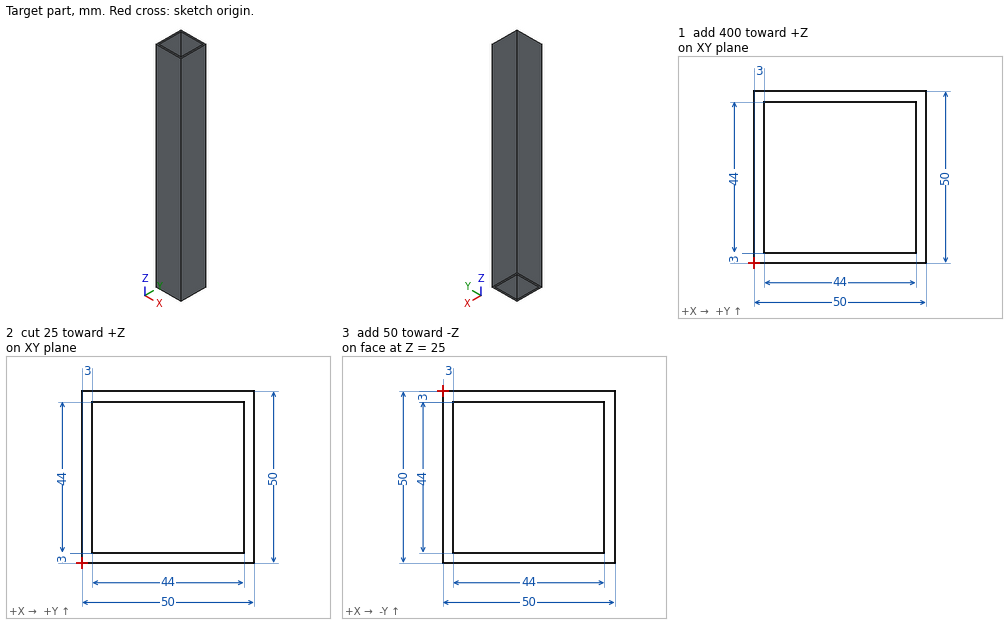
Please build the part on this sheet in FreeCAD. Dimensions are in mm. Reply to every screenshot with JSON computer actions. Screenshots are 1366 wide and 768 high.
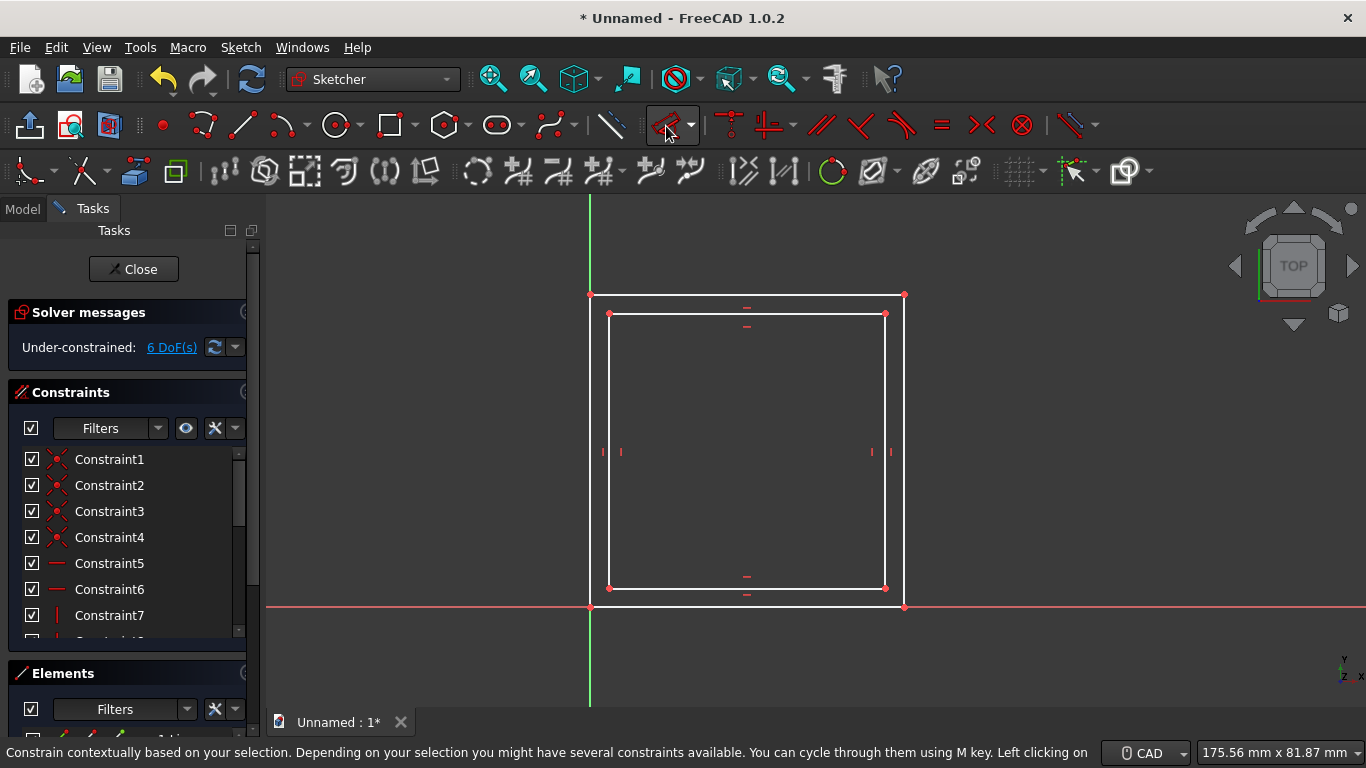
{"action": "left_click", "coordinate": [684, 607]}
{"action": "left_click", "coordinate": [747, 641]}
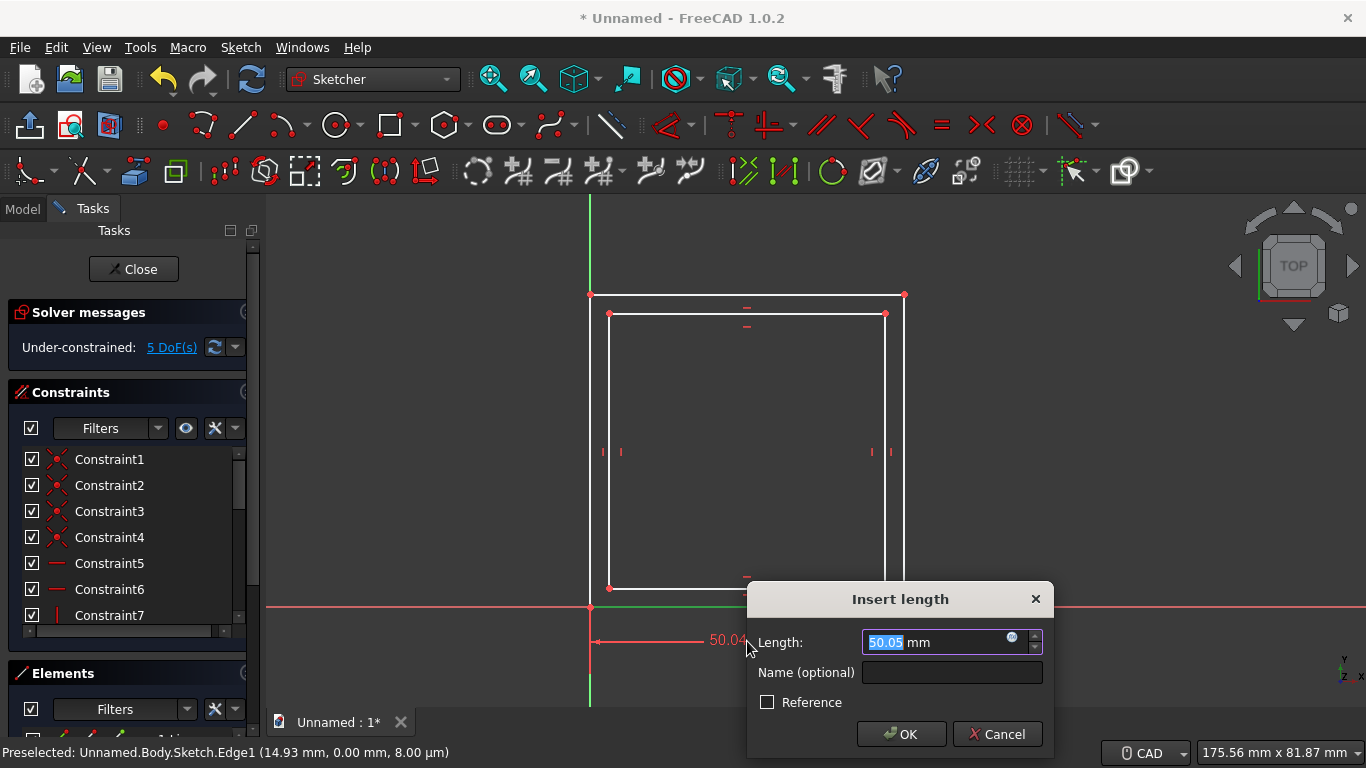
{"action": "type", "text": "50"}
{"action": "key", "text": "Return"}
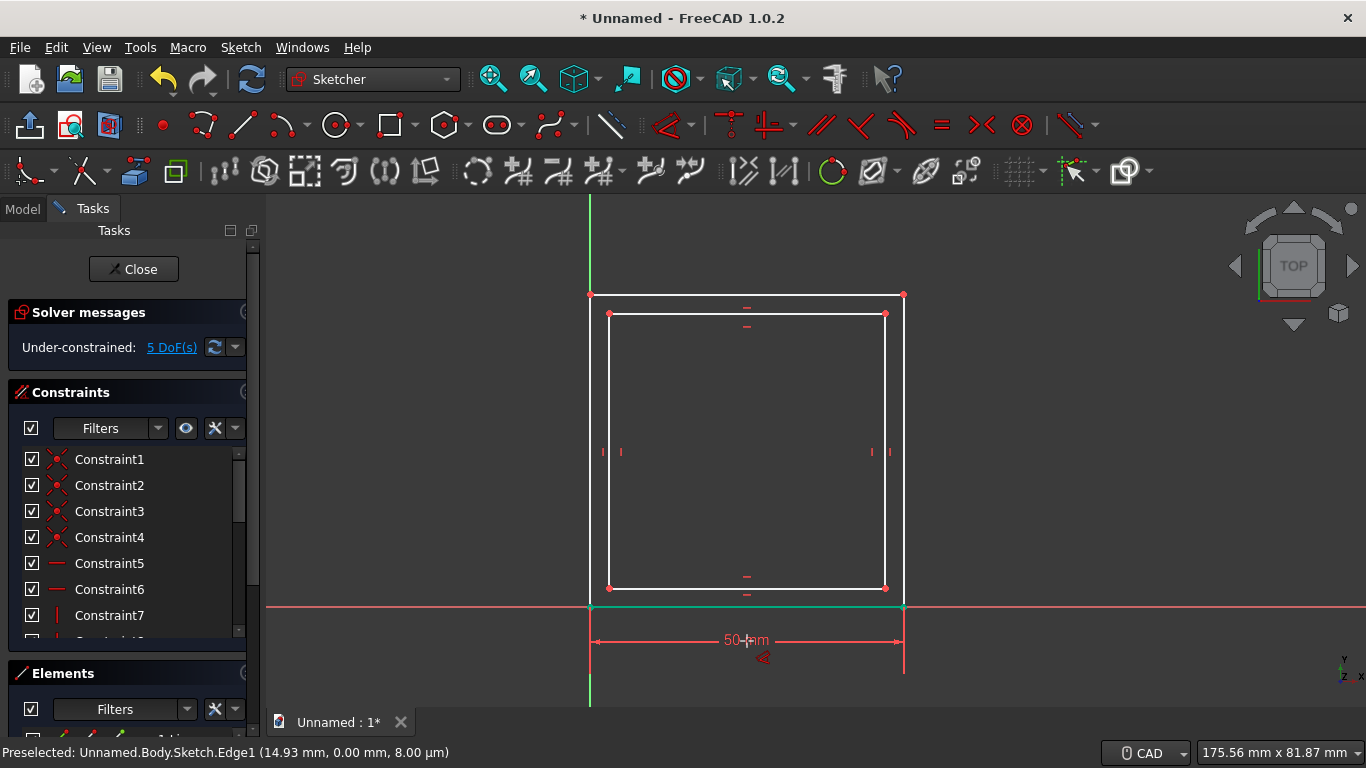
{"action": "left_click", "coordinate": [904, 514]}
{"action": "left_click", "coordinate": [938, 451]}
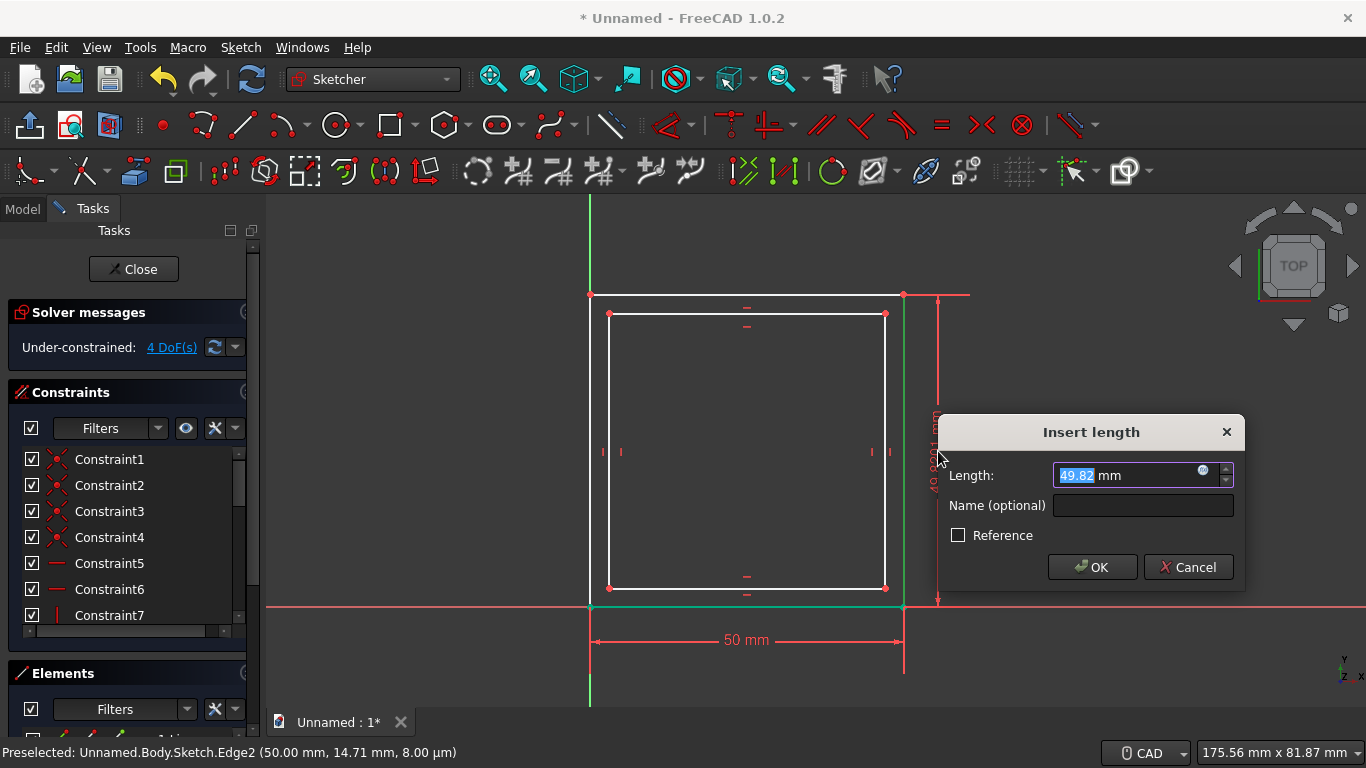
{"action": "type", "text": "50"}
{"action": "key", "text": "Return"}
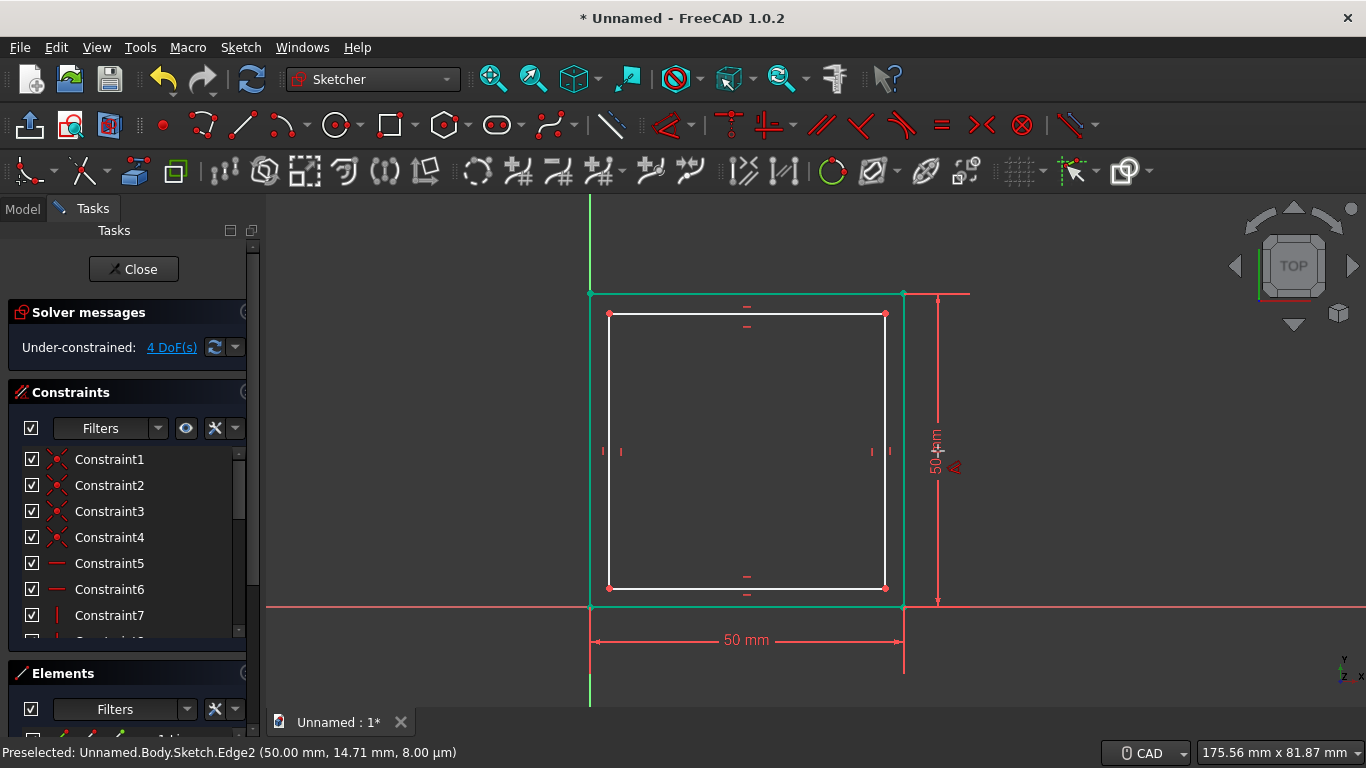
{"action": "left_click", "coordinate": [609, 396]}
{"action": "left_click", "coordinate": [575, 451]}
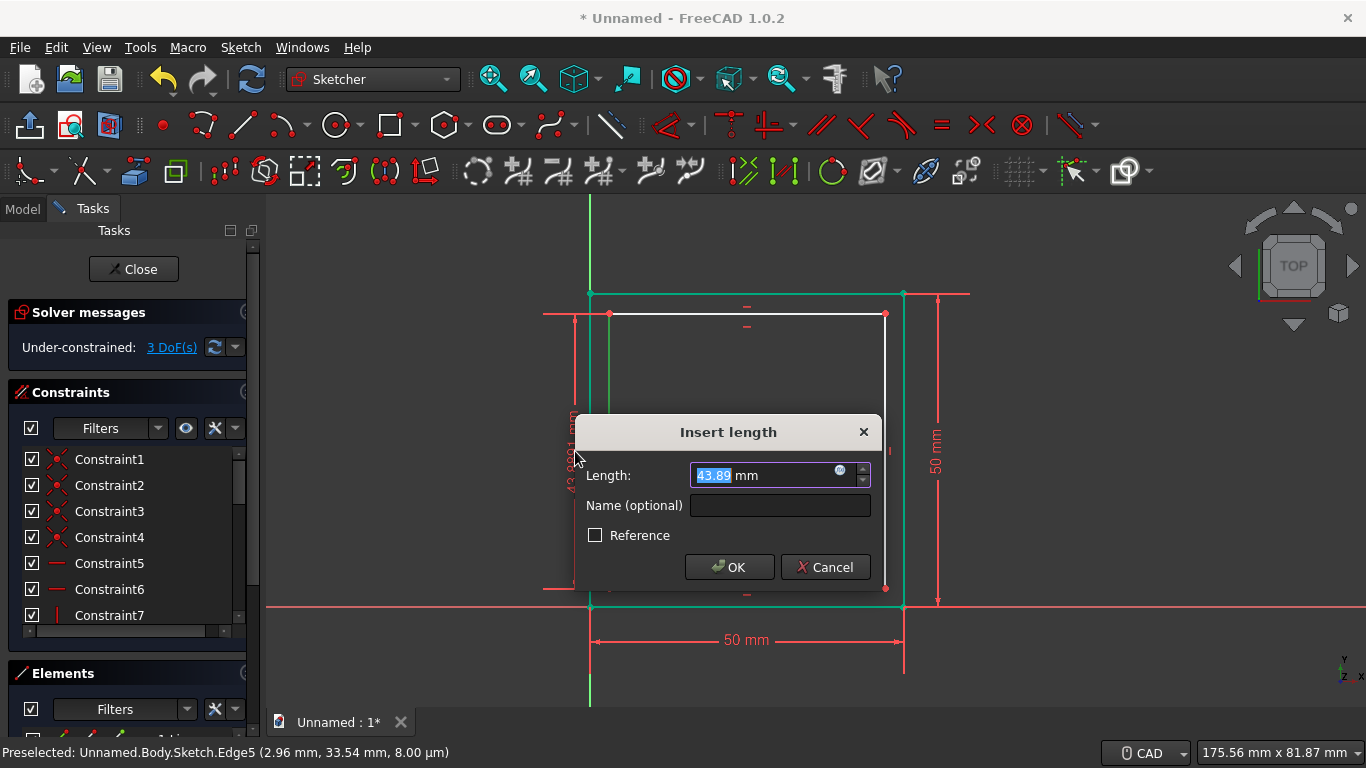
{"action": "type", "text": "44"}
{"action": "key", "text": "Return"}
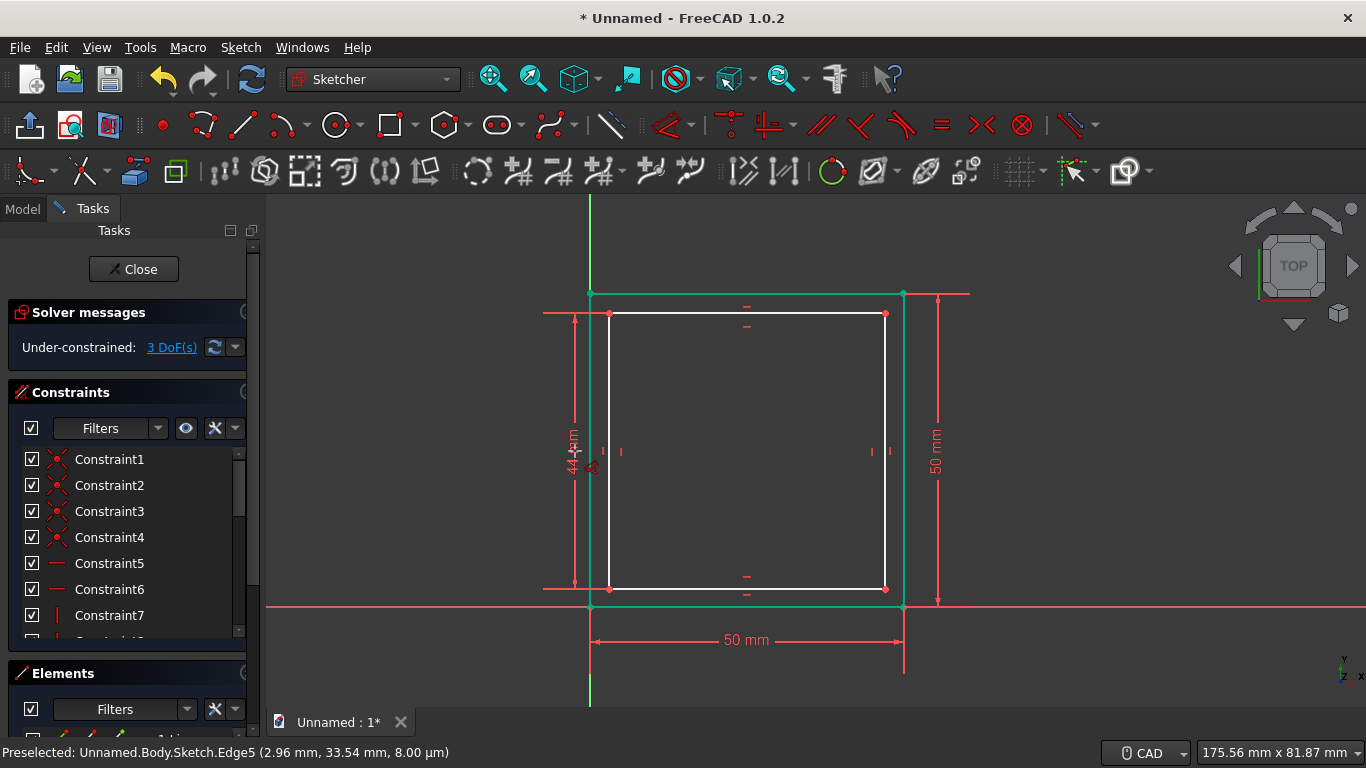
{"action": "left_click", "coordinate": [692, 589]}
{"action": "left_click", "coordinate": [650, 623]}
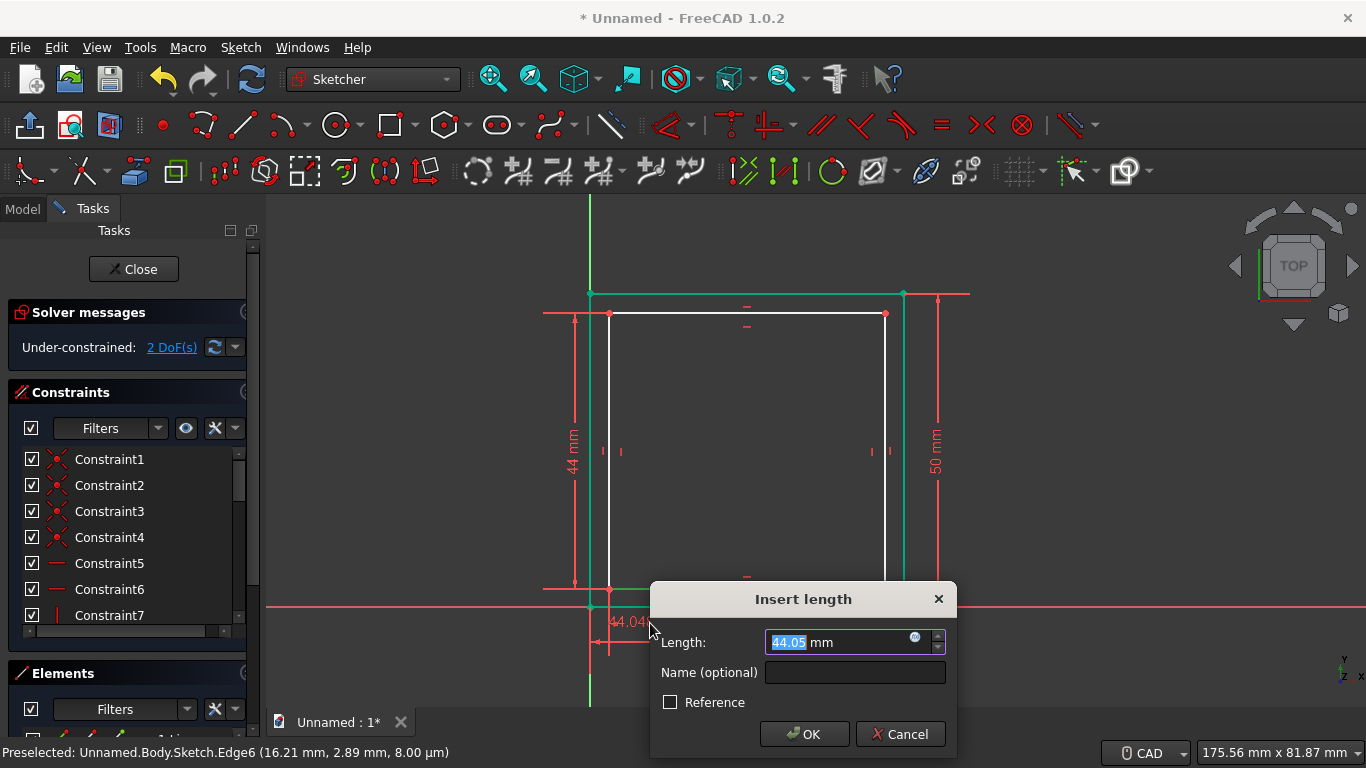
{"action": "type", "text": "44"}
{"action": "key", "text": "Return"}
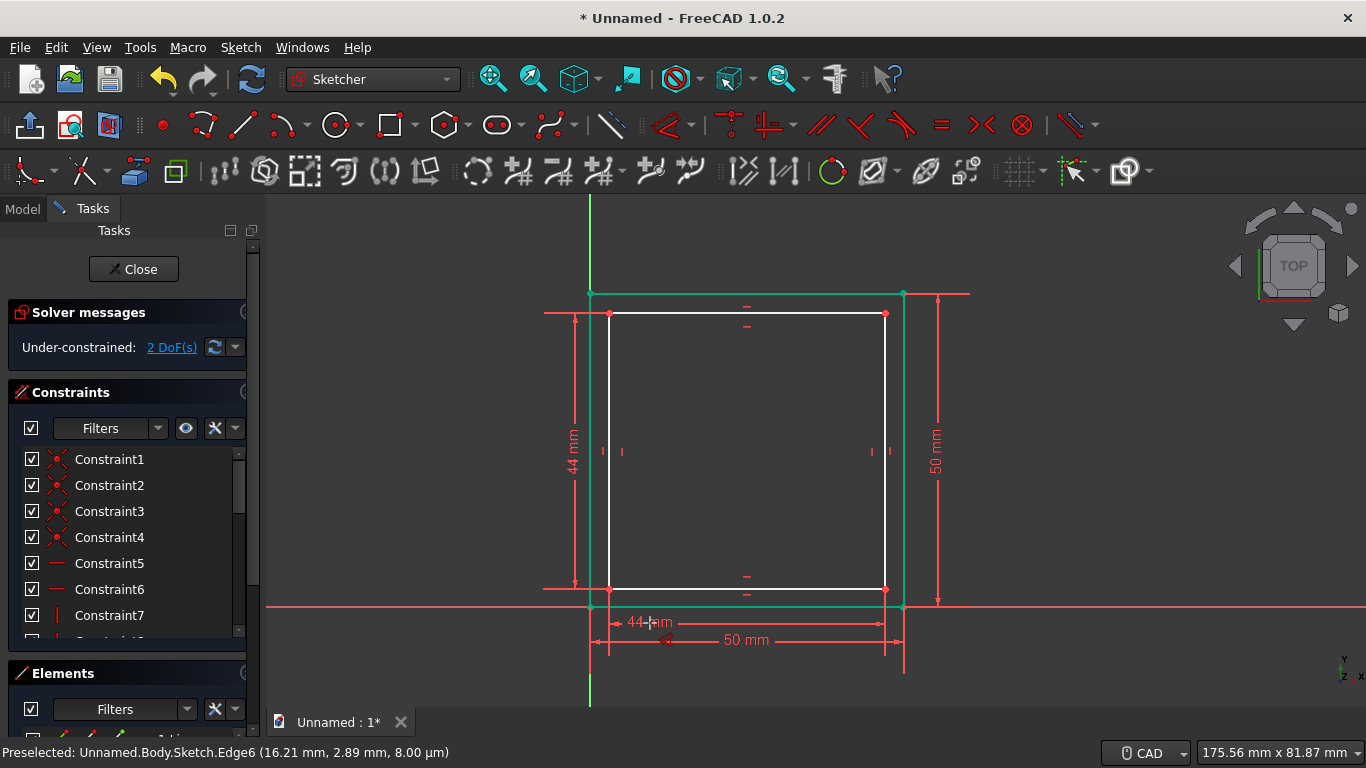
{"action": "scroll", "coordinate": [609, 313], "scroll_direction": "up", "scroll_amount": 4}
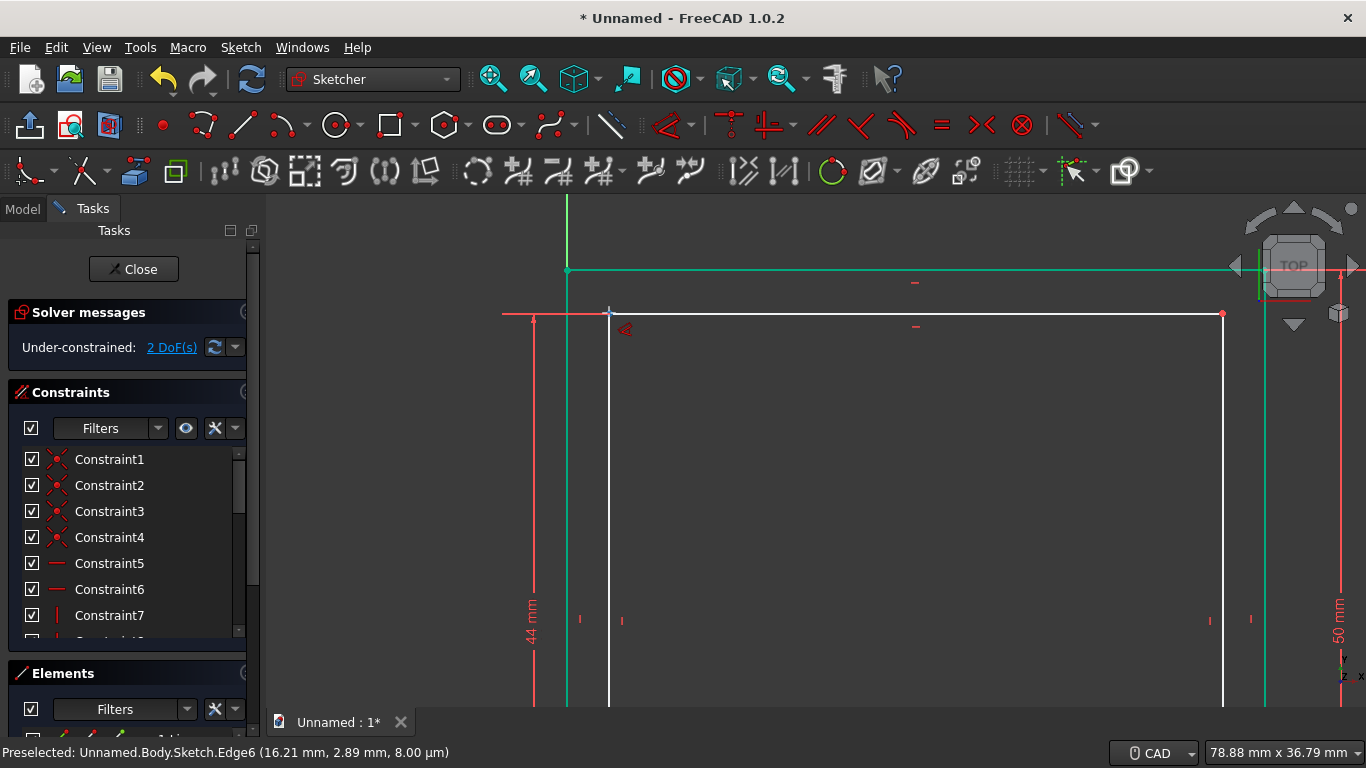
{"action": "left_click", "coordinate": [609, 314]}
{"action": "left_click", "coordinate": [588, 256]}